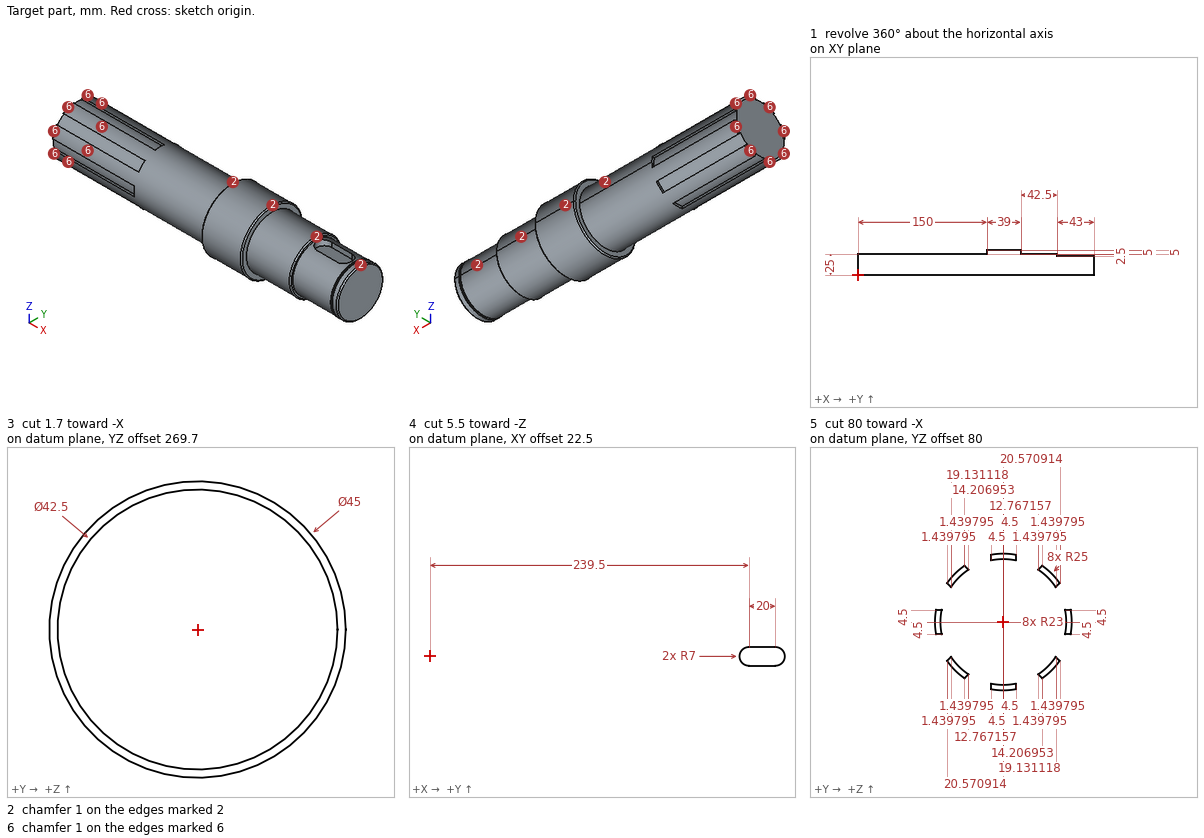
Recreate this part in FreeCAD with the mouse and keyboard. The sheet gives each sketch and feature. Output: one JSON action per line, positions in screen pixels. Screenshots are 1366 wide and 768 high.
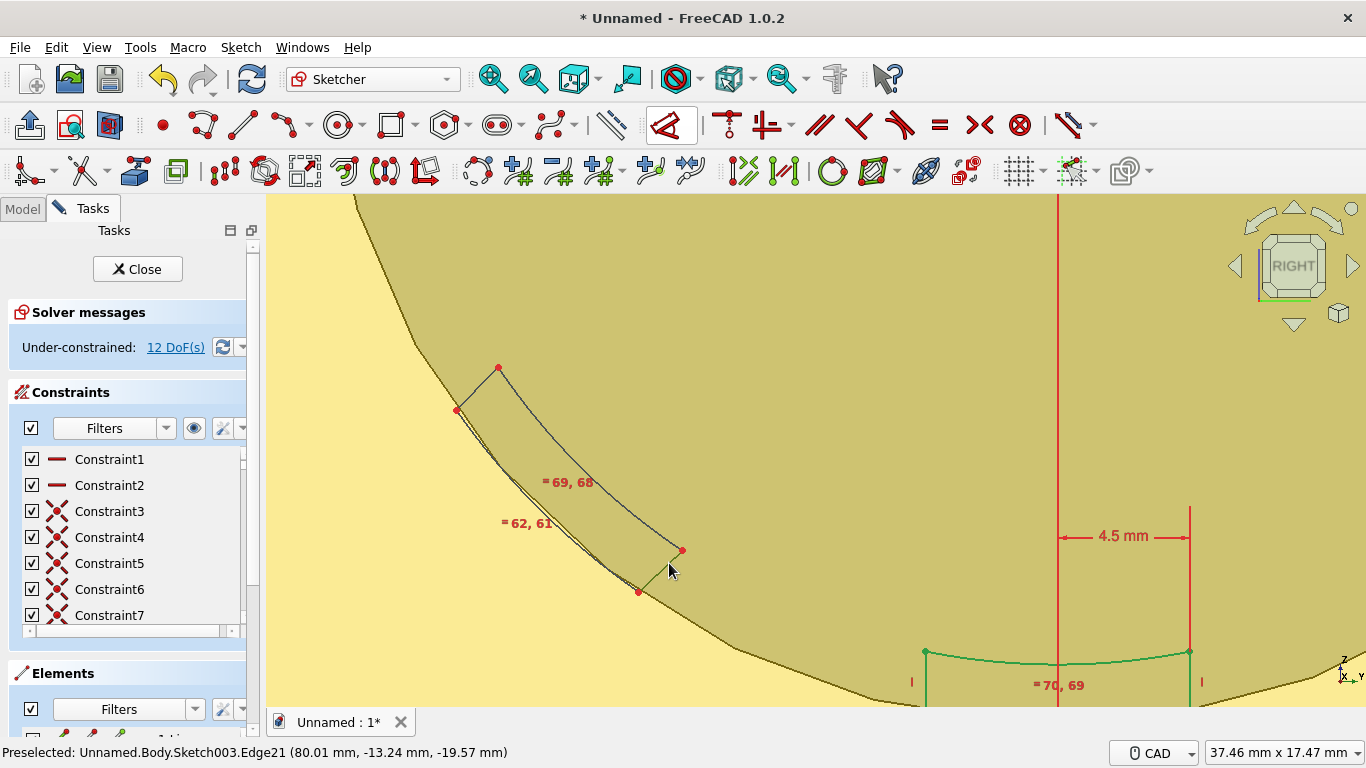
{"action": "left_click", "coordinate": [692, 126]}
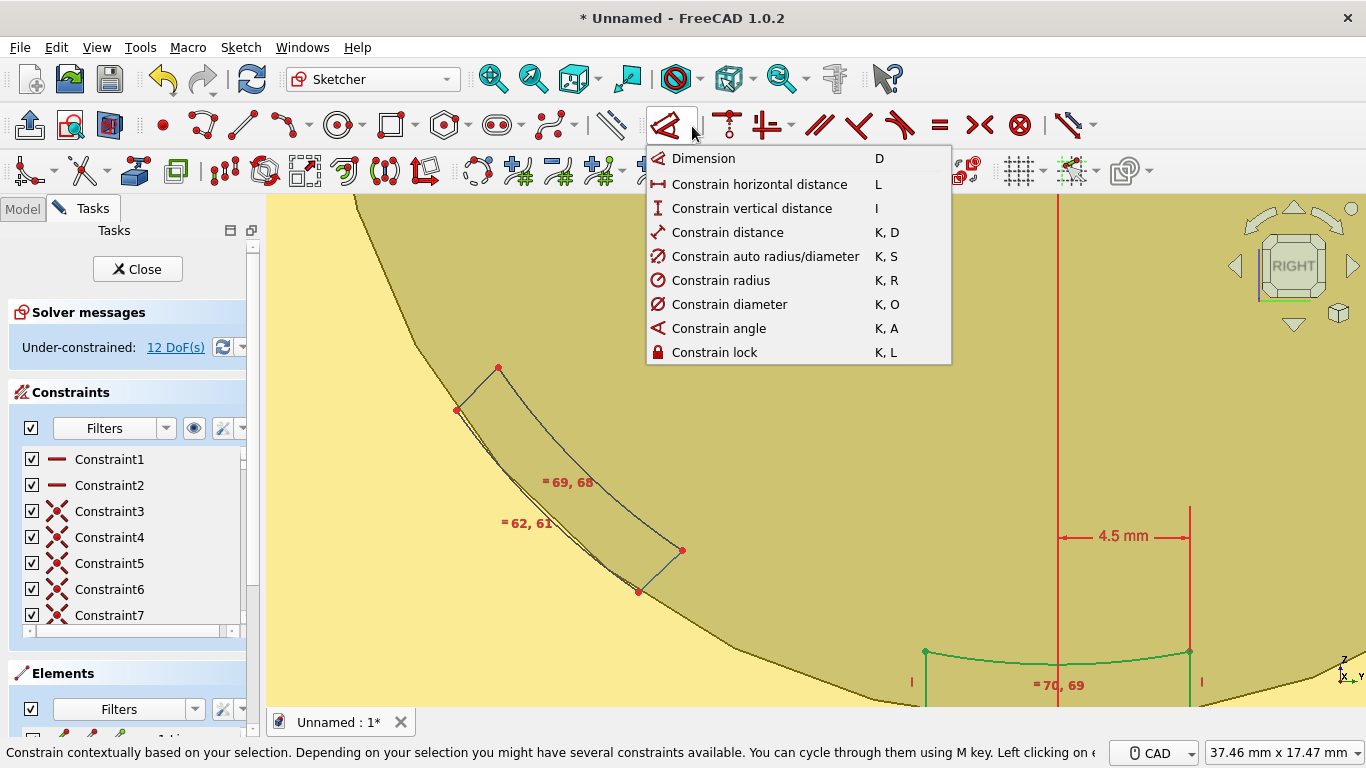
{"action": "left_click", "coordinate": [799, 184]}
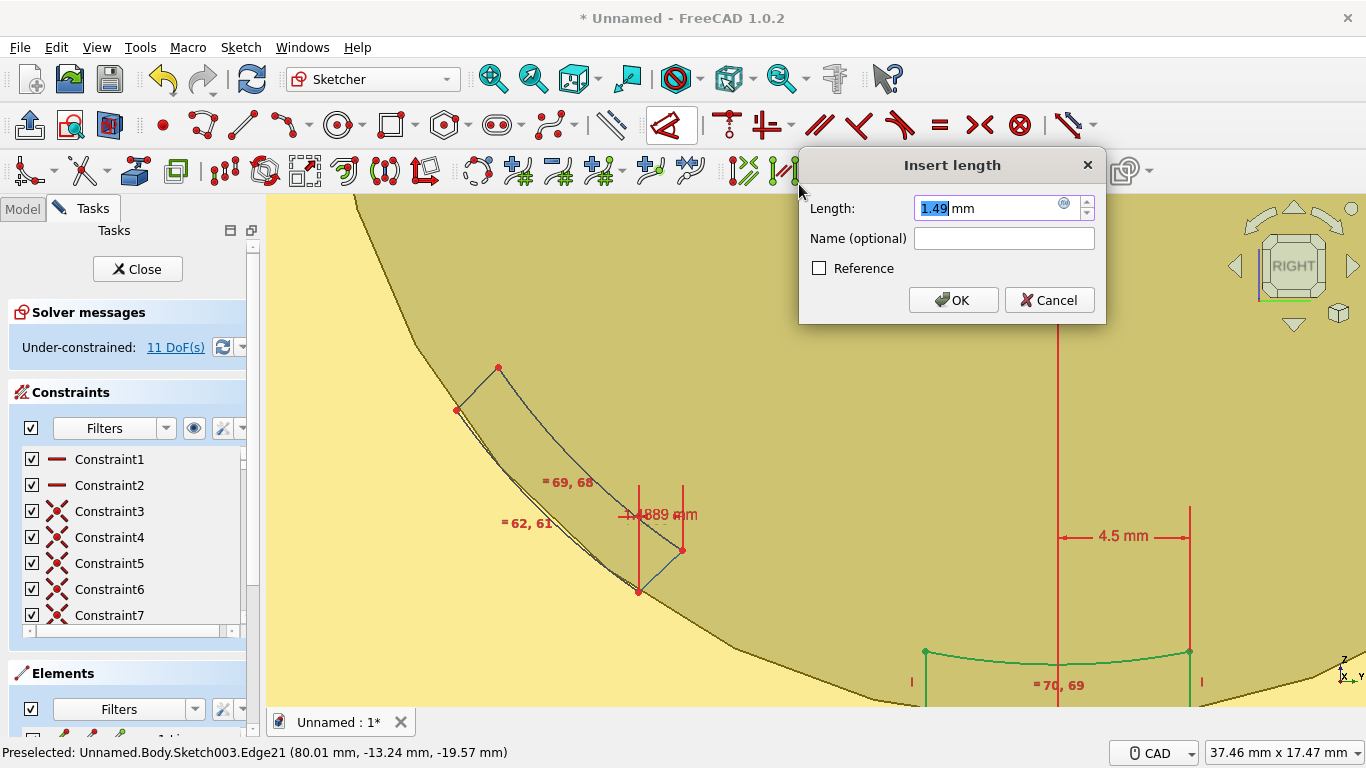
{"action": "type", "text": "1.439795"}
{"action": "key", "text": "Return"}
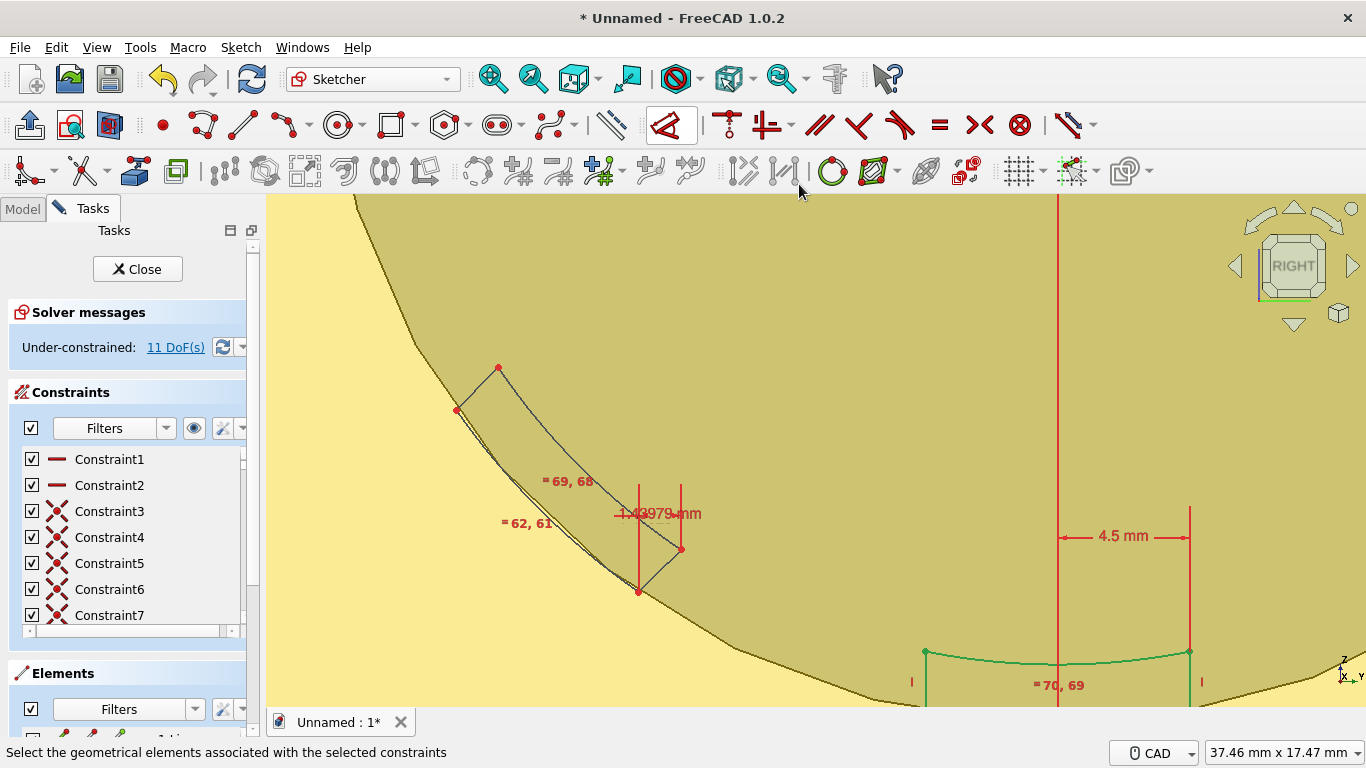
{"action": "left_click", "coordinate": [469, 397]}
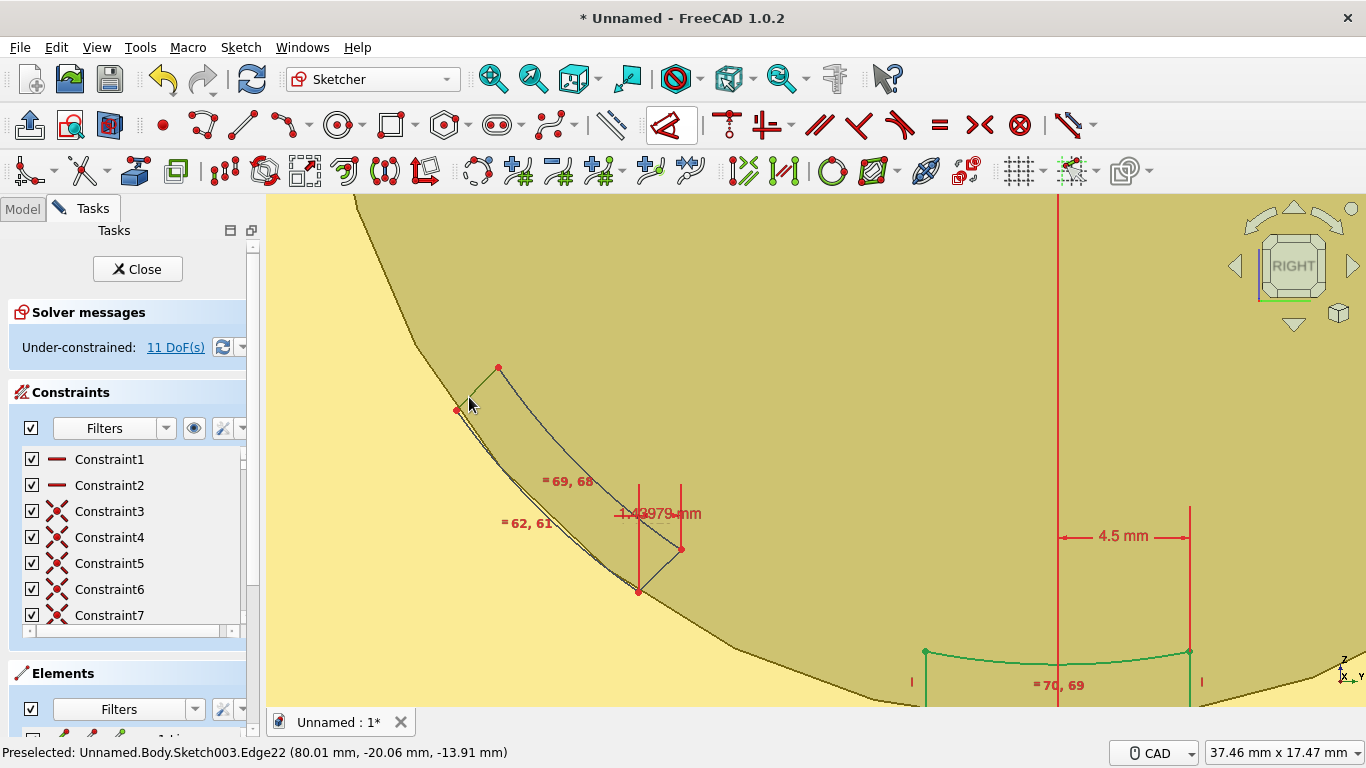
{"action": "key", "text": "l"}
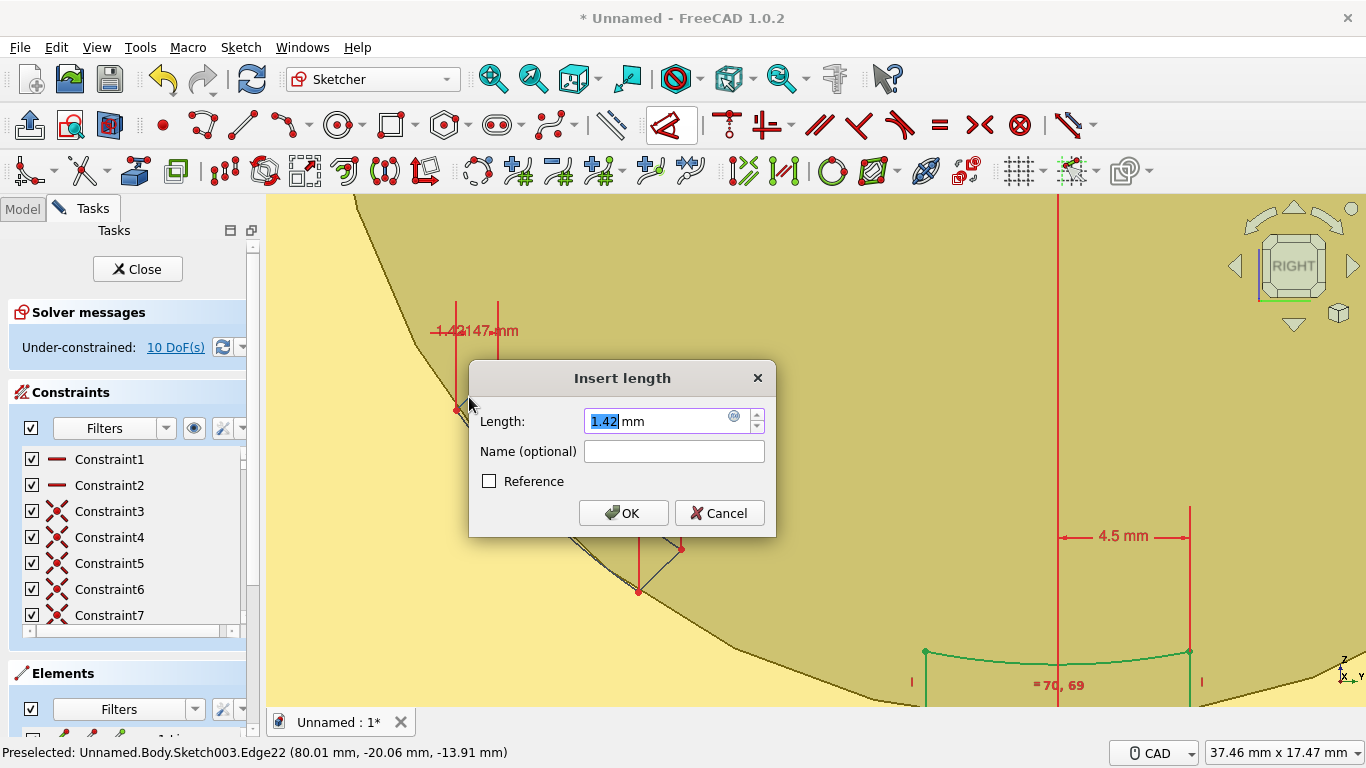
{"action": "type", "text": "1.439795"}
{"action": "key", "text": "Return"}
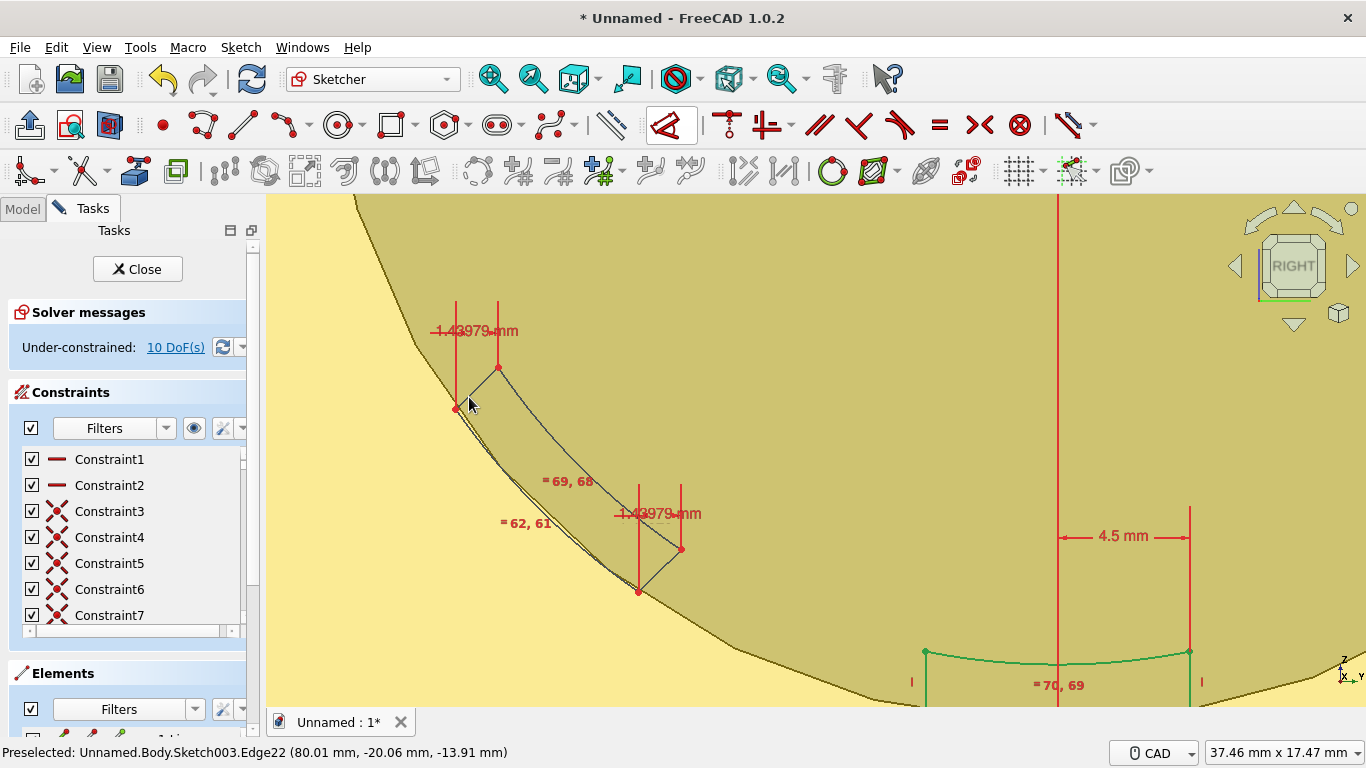
{"action": "scroll", "coordinate": [669, 567], "scroll_direction": "down", "scroll_amount": 8}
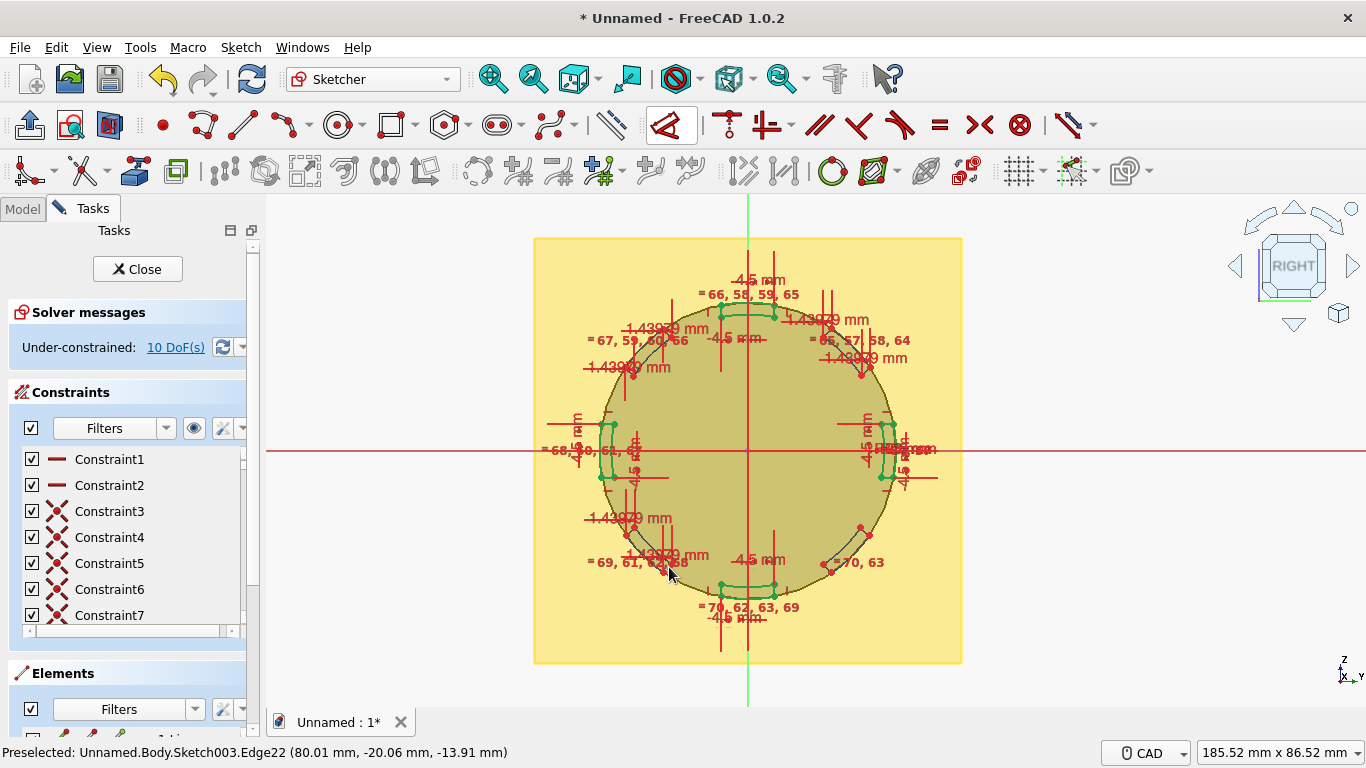
{"action": "scroll", "coordinate": [863, 530], "scroll_direction": "up", "scroll_amount": 8}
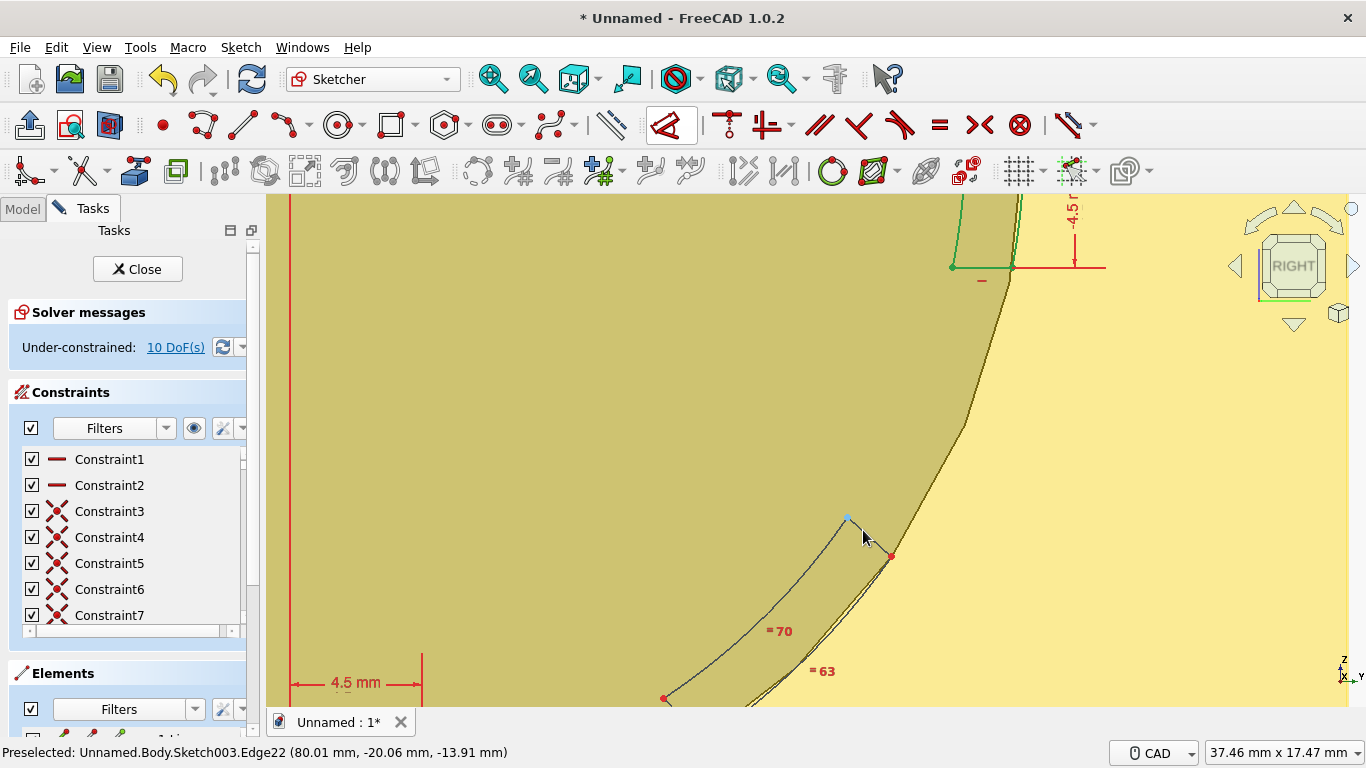
{"action": "left_click", "coordinate": [861, 529]}